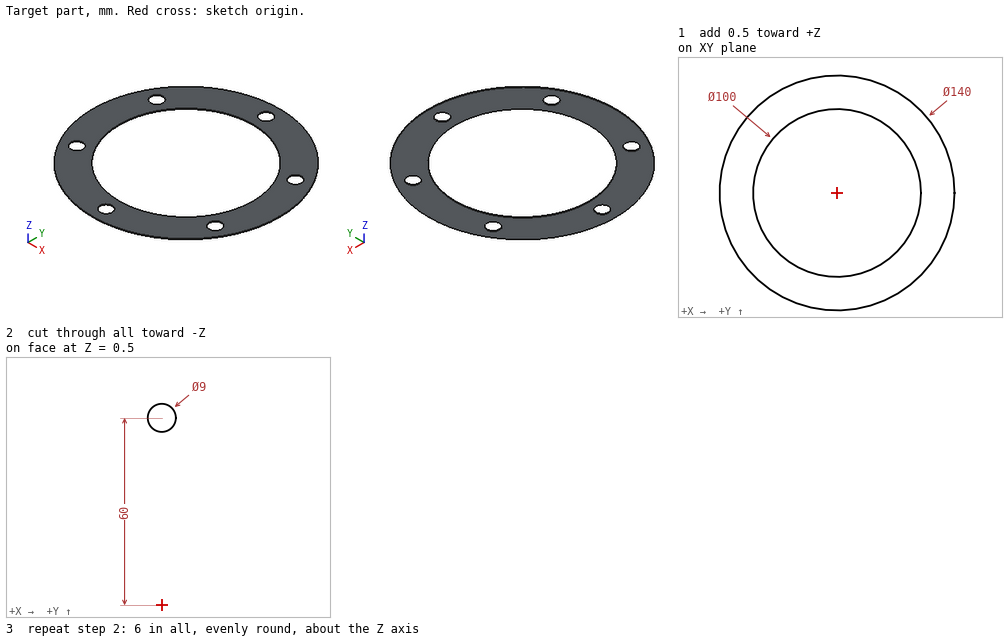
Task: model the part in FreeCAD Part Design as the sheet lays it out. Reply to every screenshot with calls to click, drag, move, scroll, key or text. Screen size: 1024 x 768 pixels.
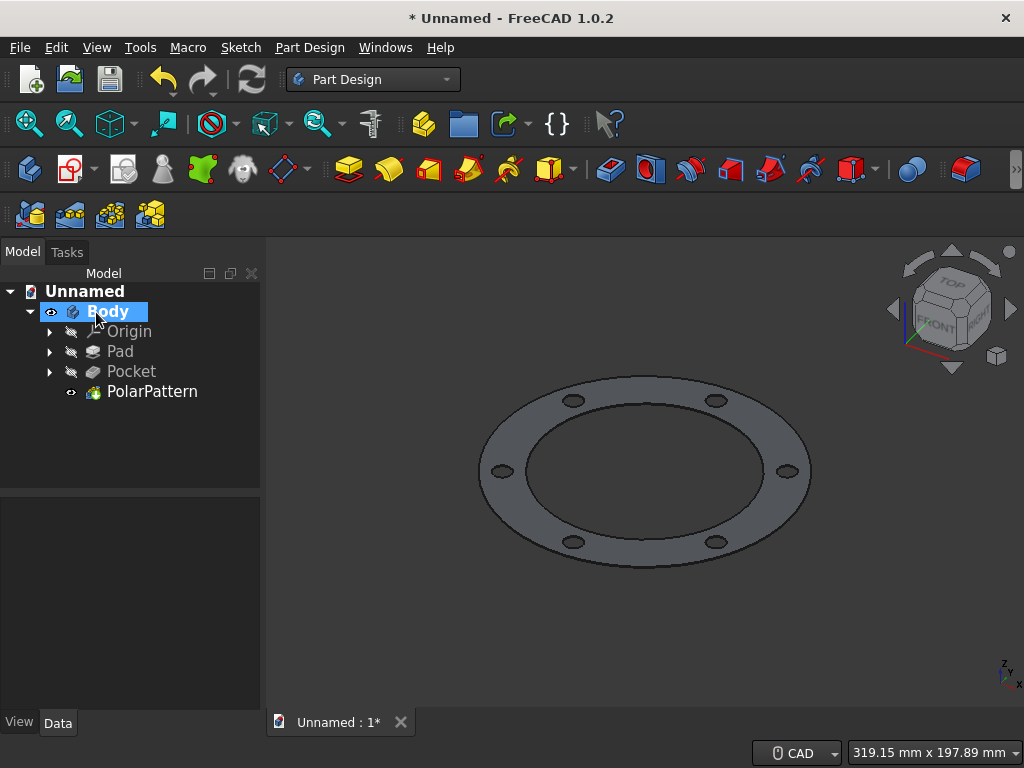
key(0)